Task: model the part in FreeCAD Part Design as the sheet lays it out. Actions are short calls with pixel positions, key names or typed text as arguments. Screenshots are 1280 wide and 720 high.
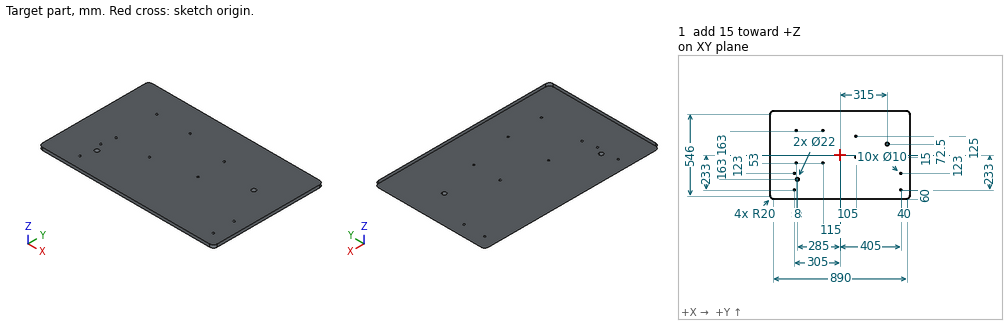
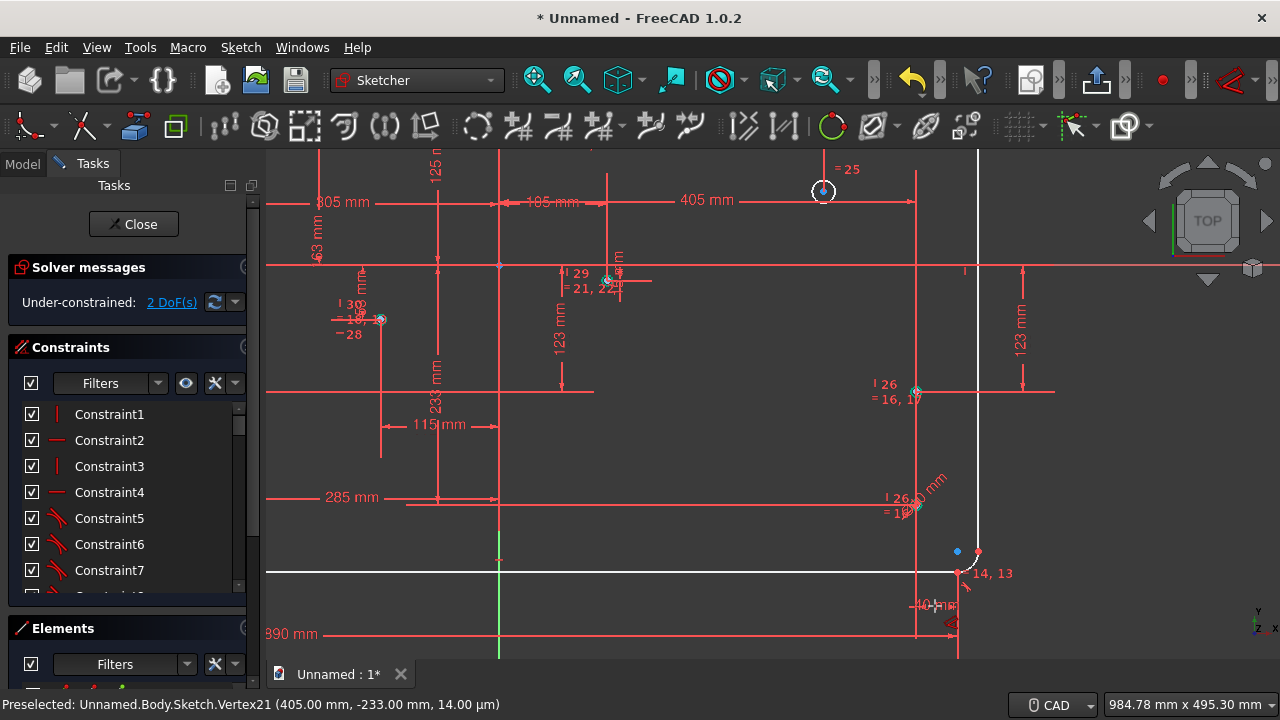
click(958, 572)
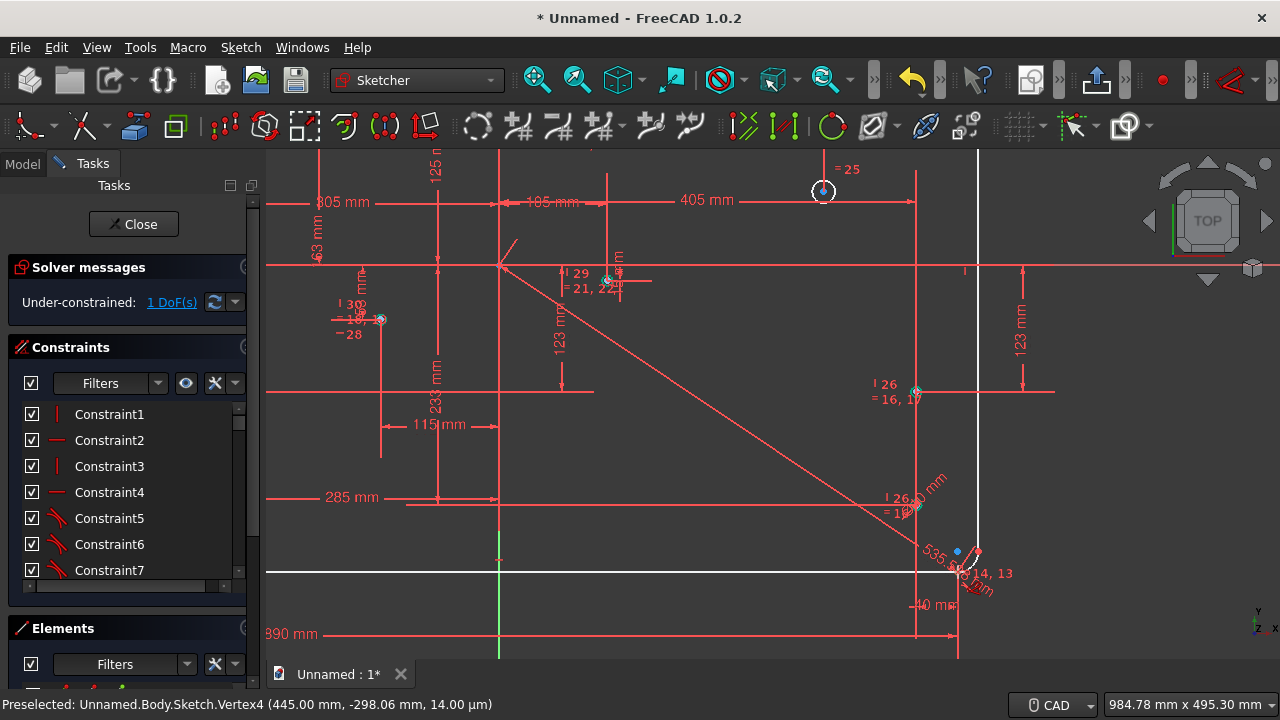
click(916, 505)
click(992, 539)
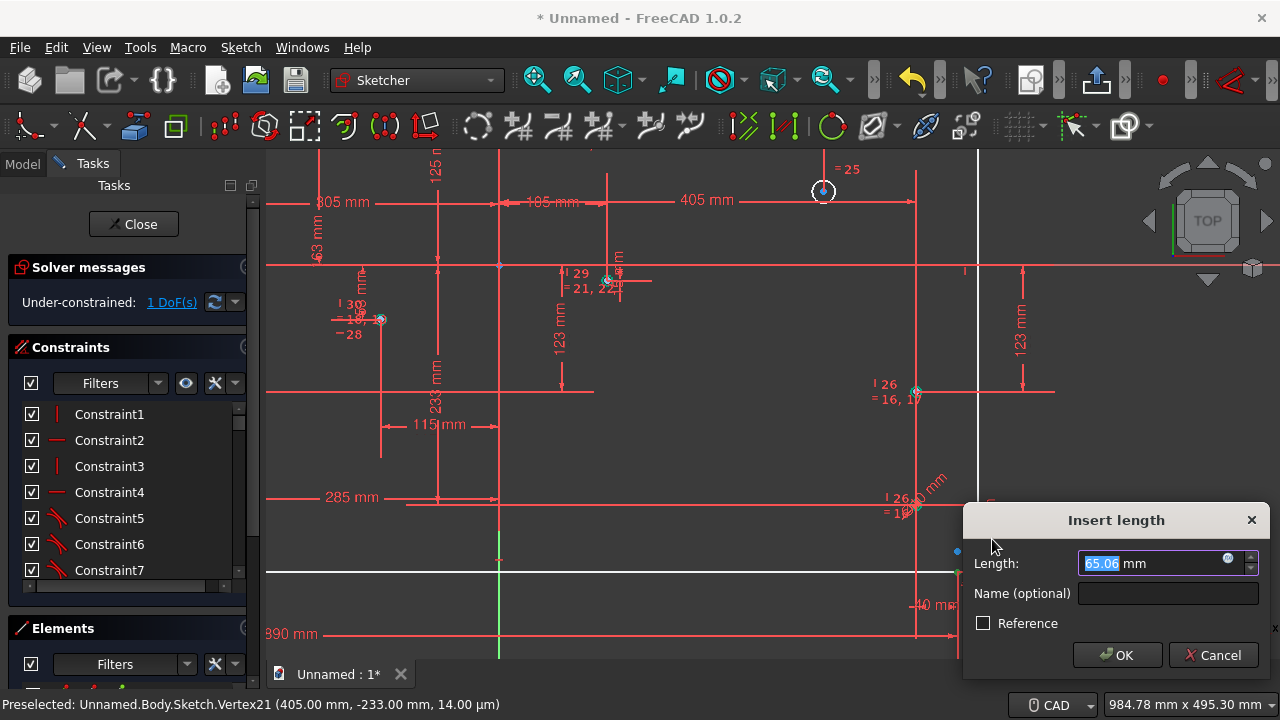
text(60)
key(Return)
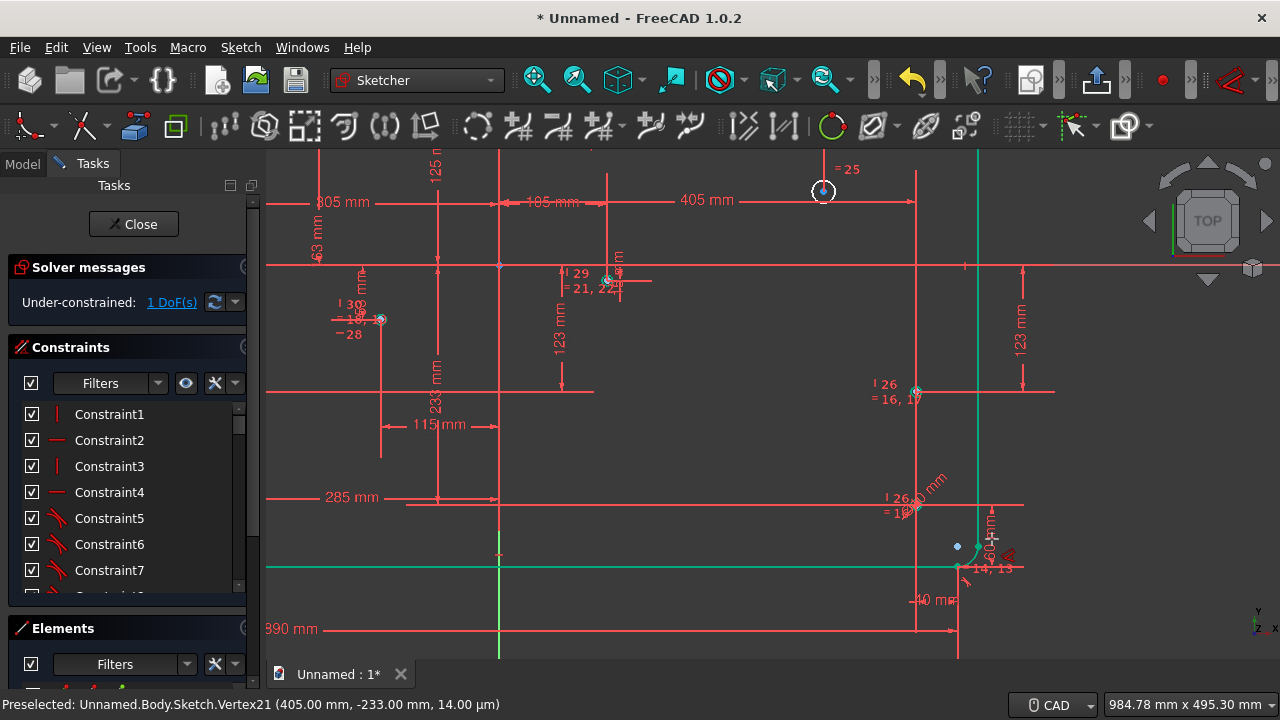
click(824, 192)
click(858, 228)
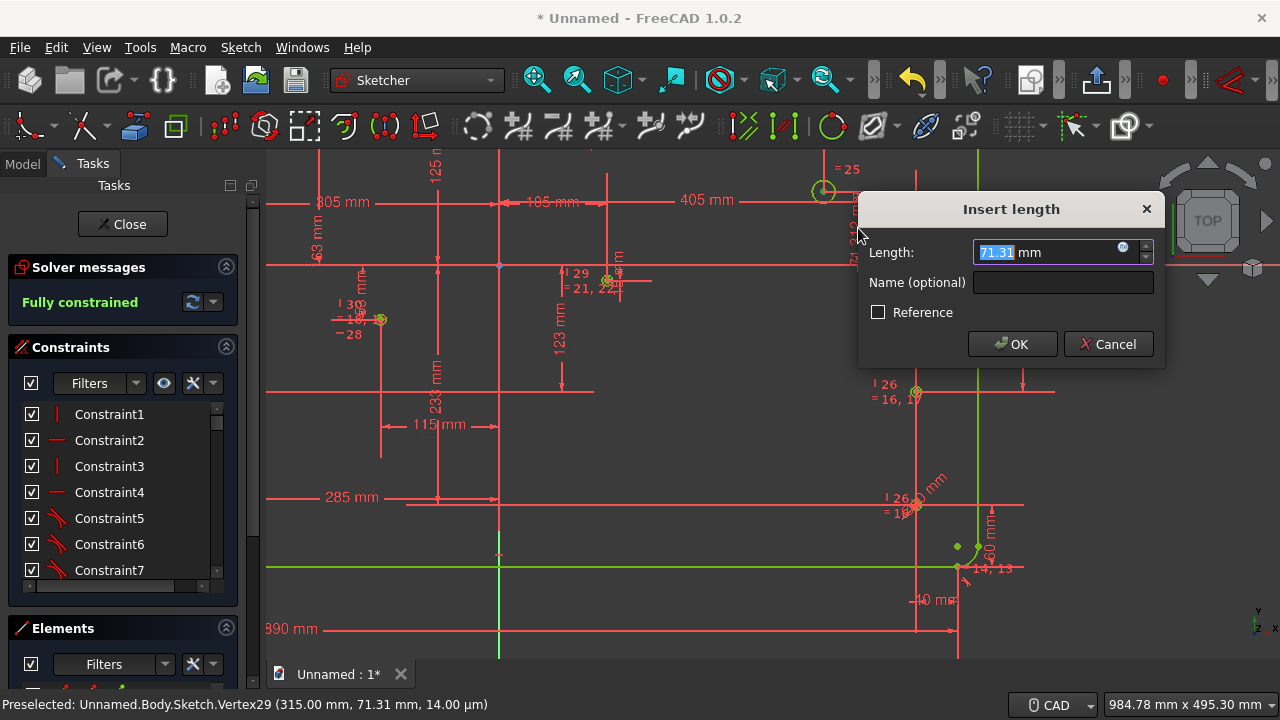
text(72.5)
key(Return)
key(Escape)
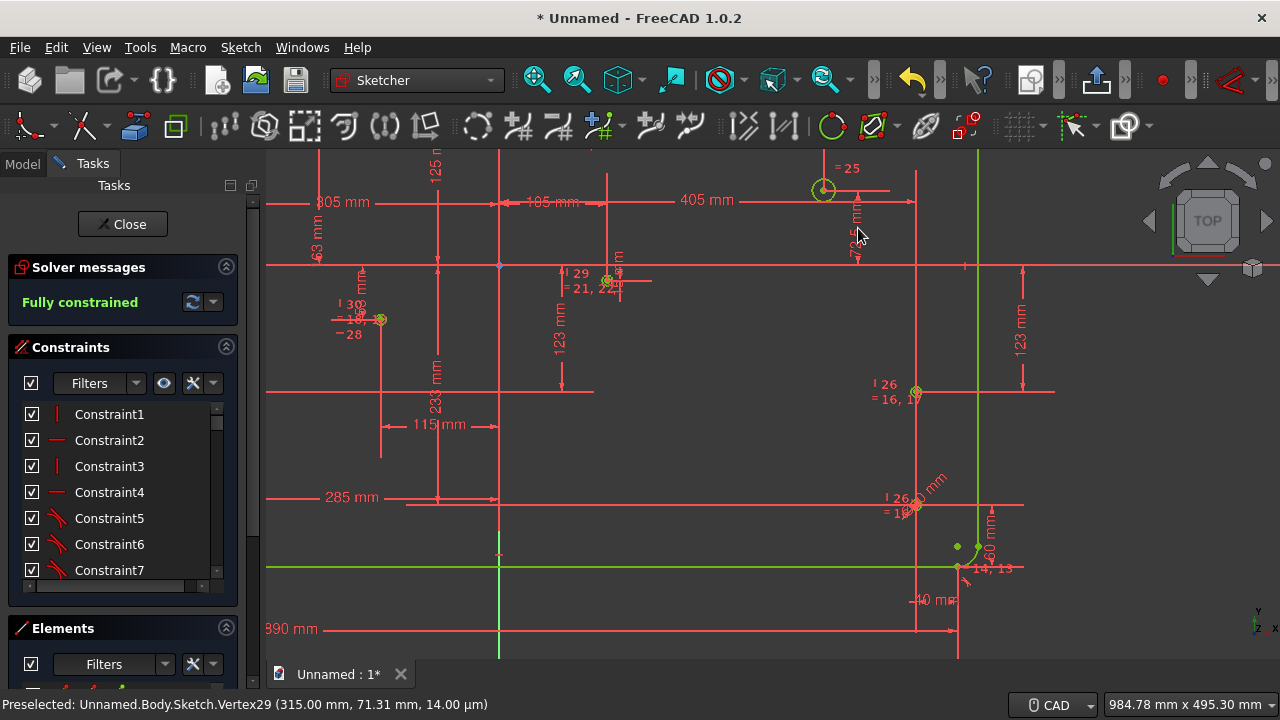
click(123, 224)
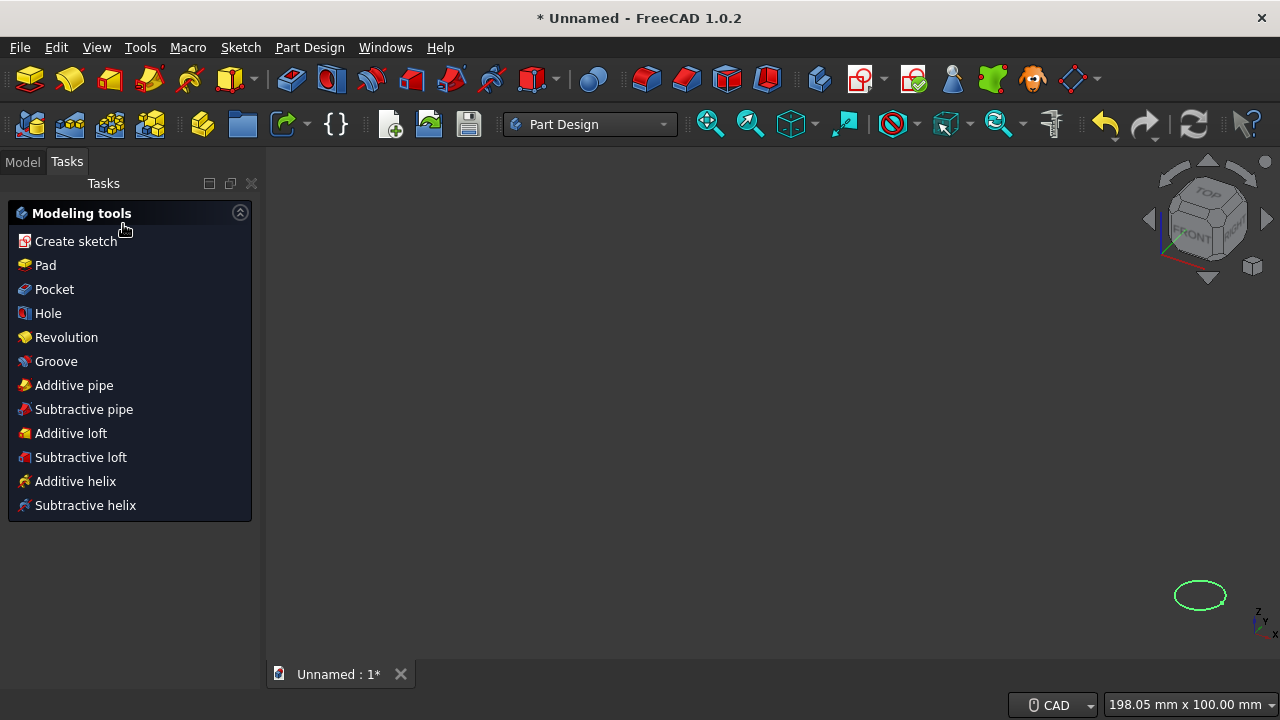
click(30, 80)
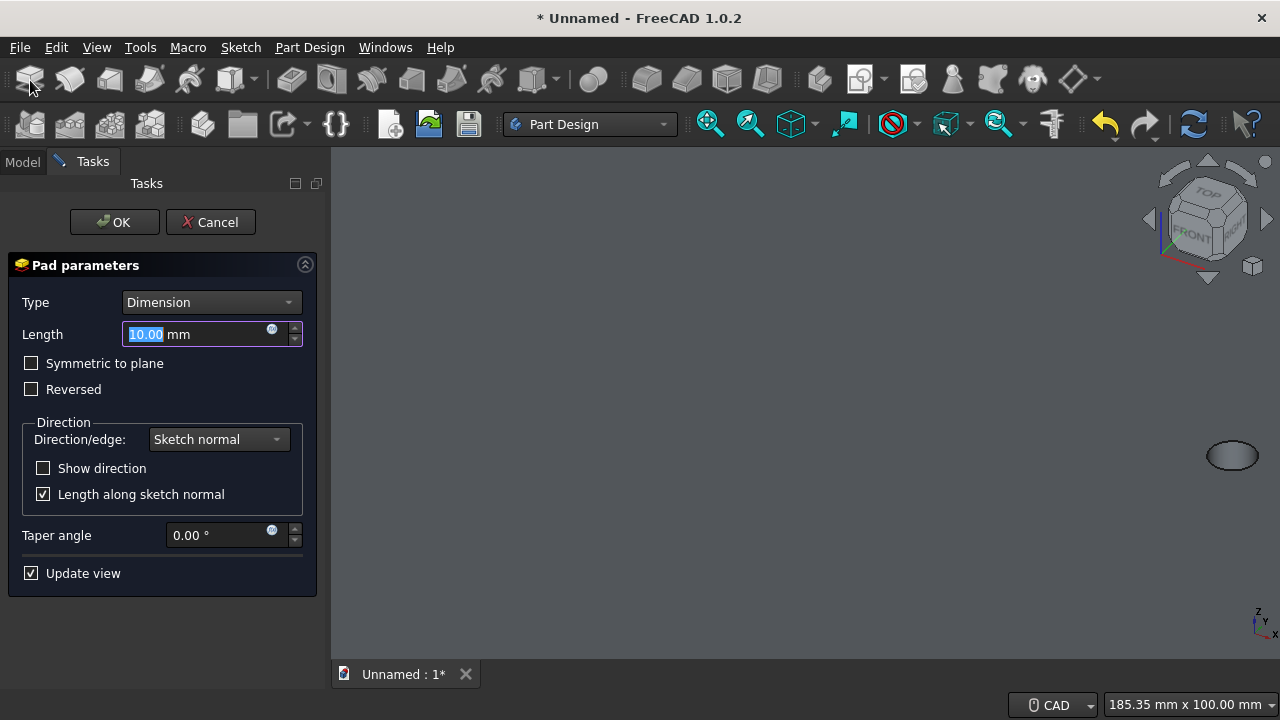
text(15)
key(Tab)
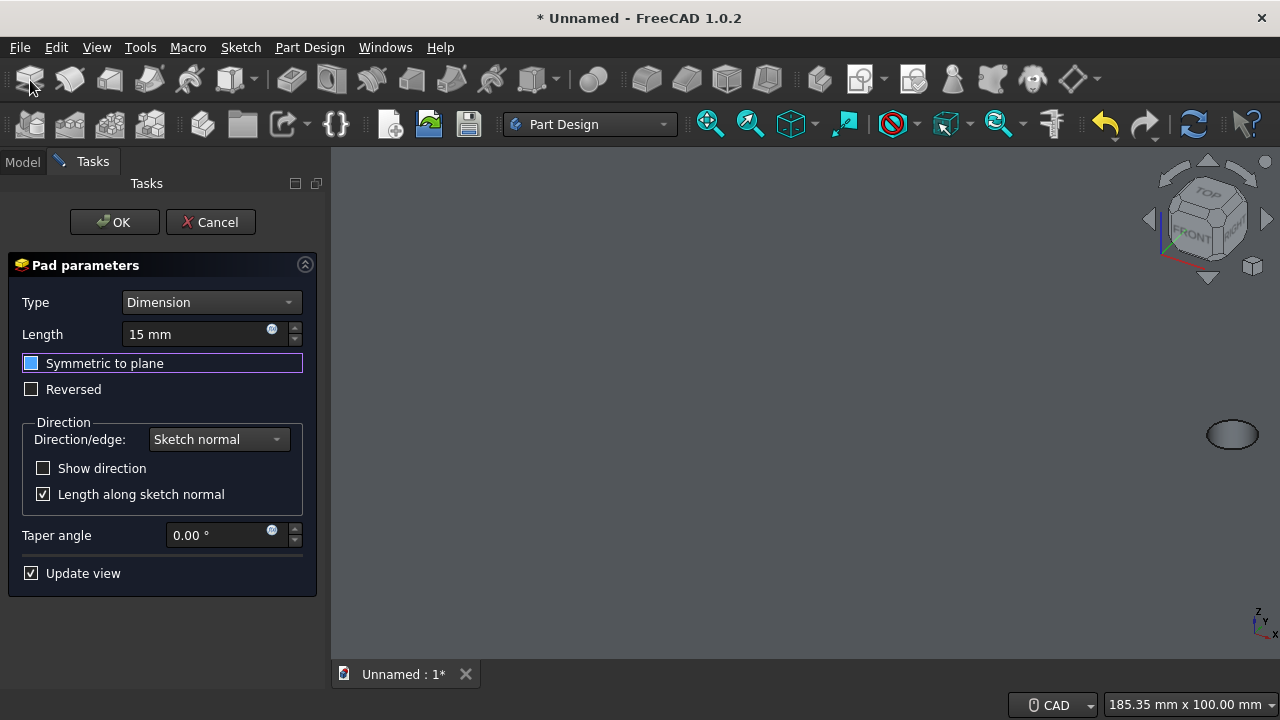
click(115, 222)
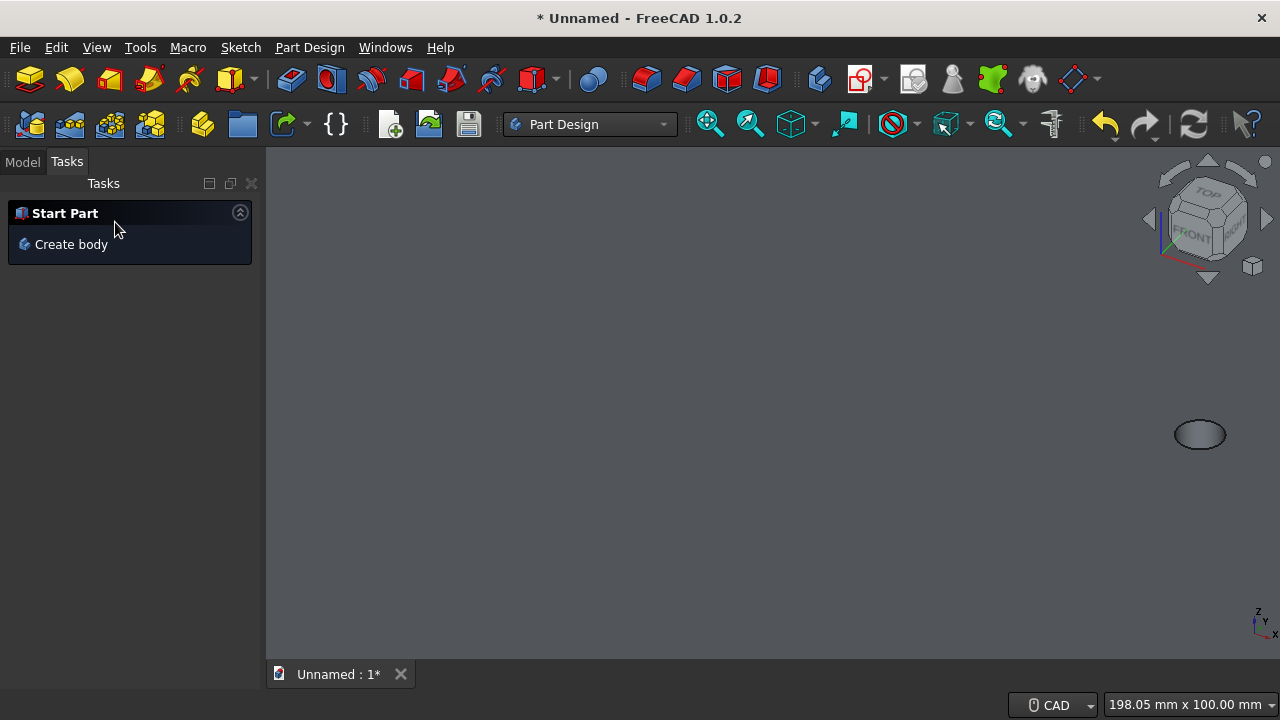
key(0)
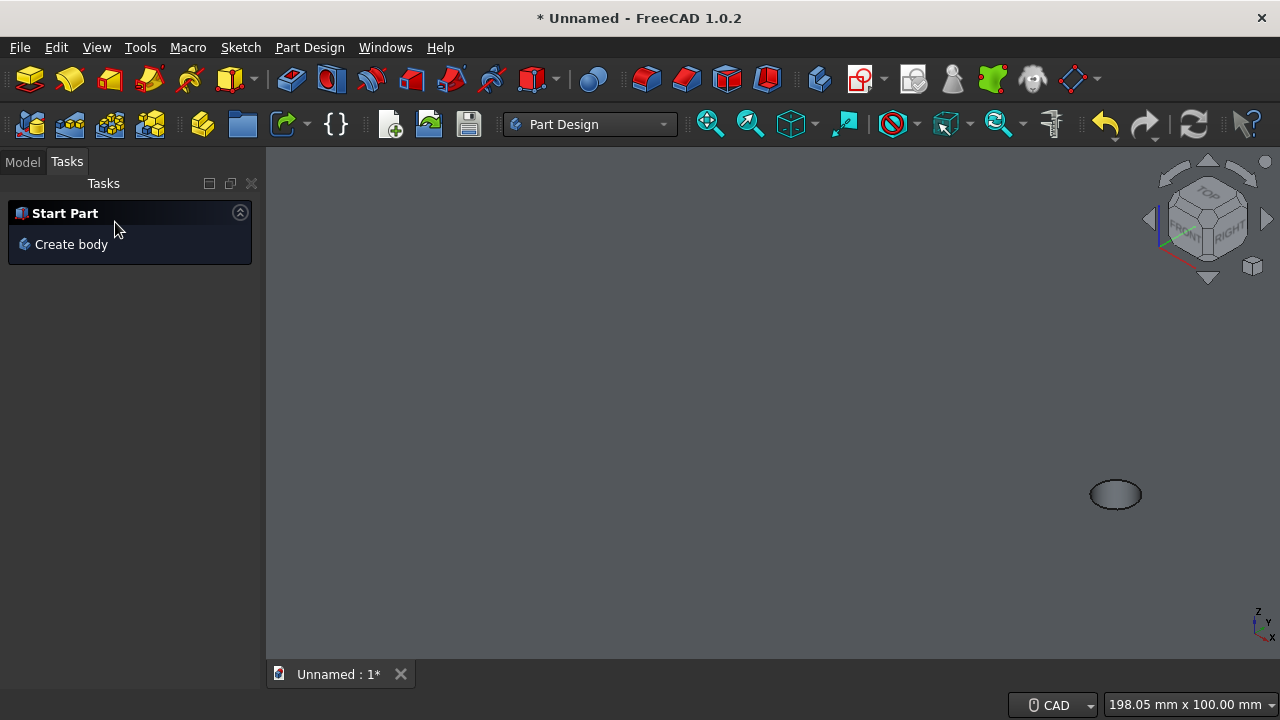
click(712, 124)